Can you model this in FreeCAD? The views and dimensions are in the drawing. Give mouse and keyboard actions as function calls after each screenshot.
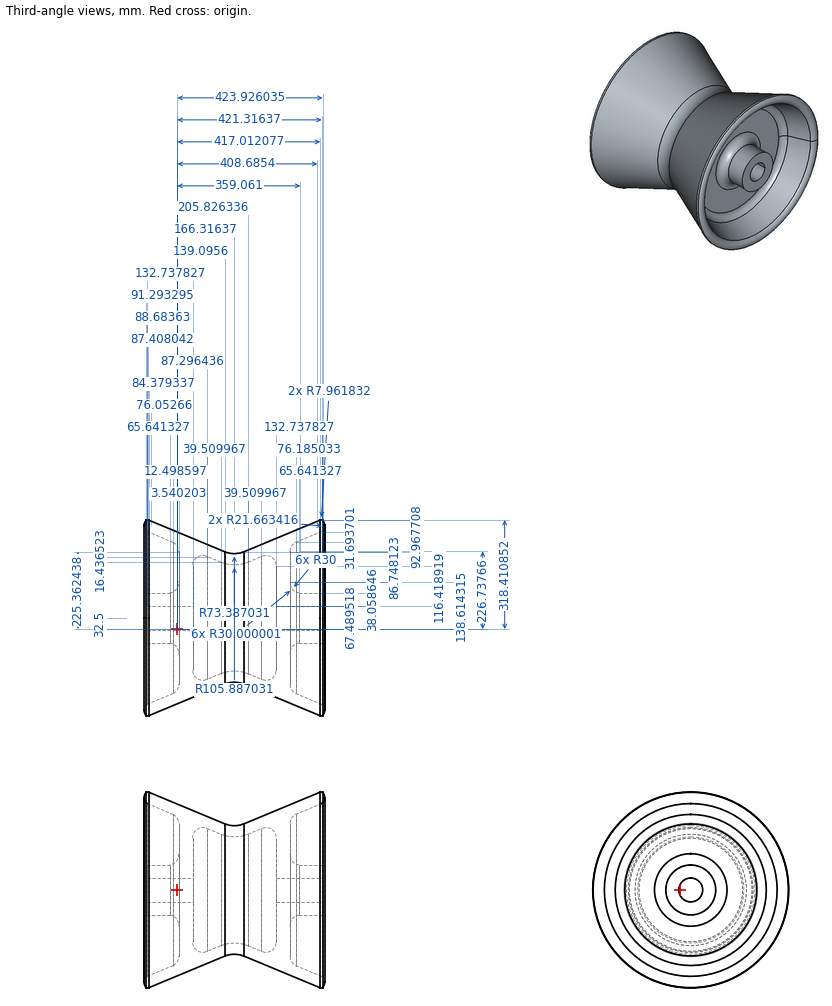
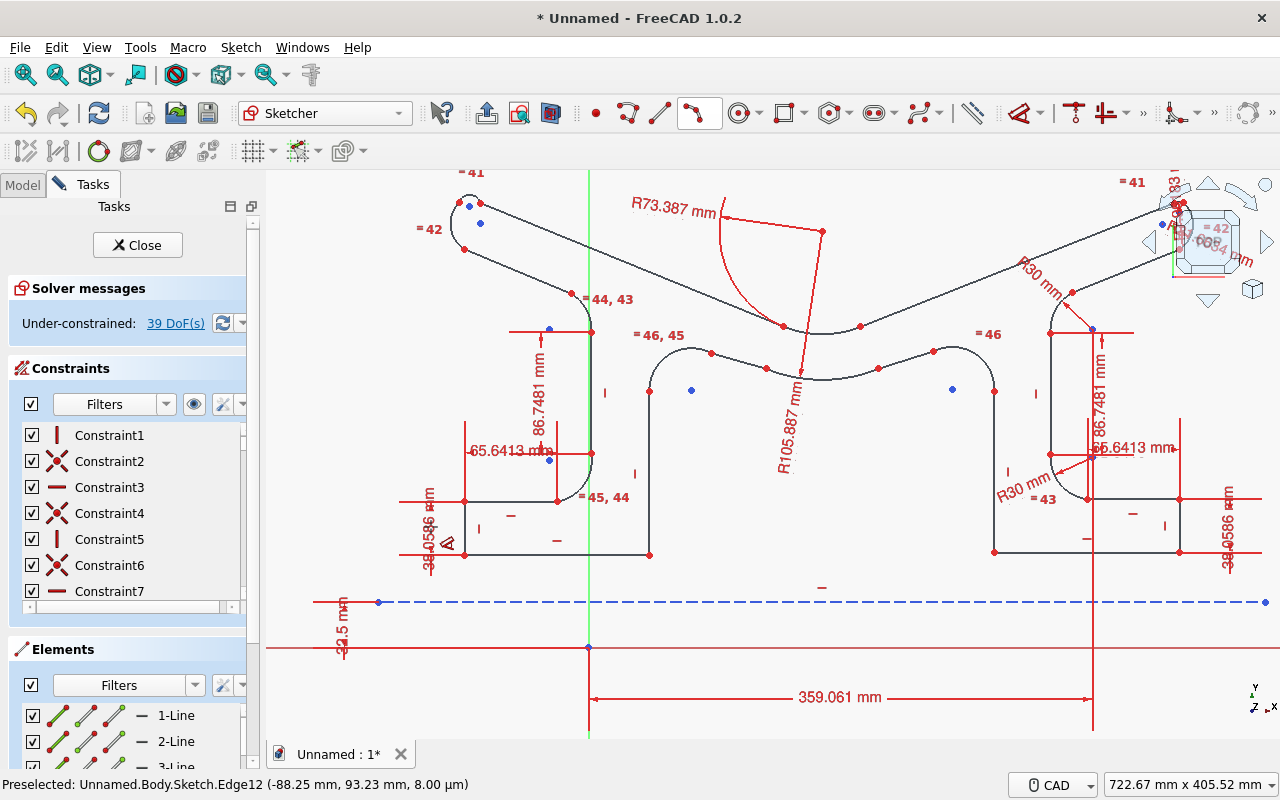
click(783, 326)
click(686, 682)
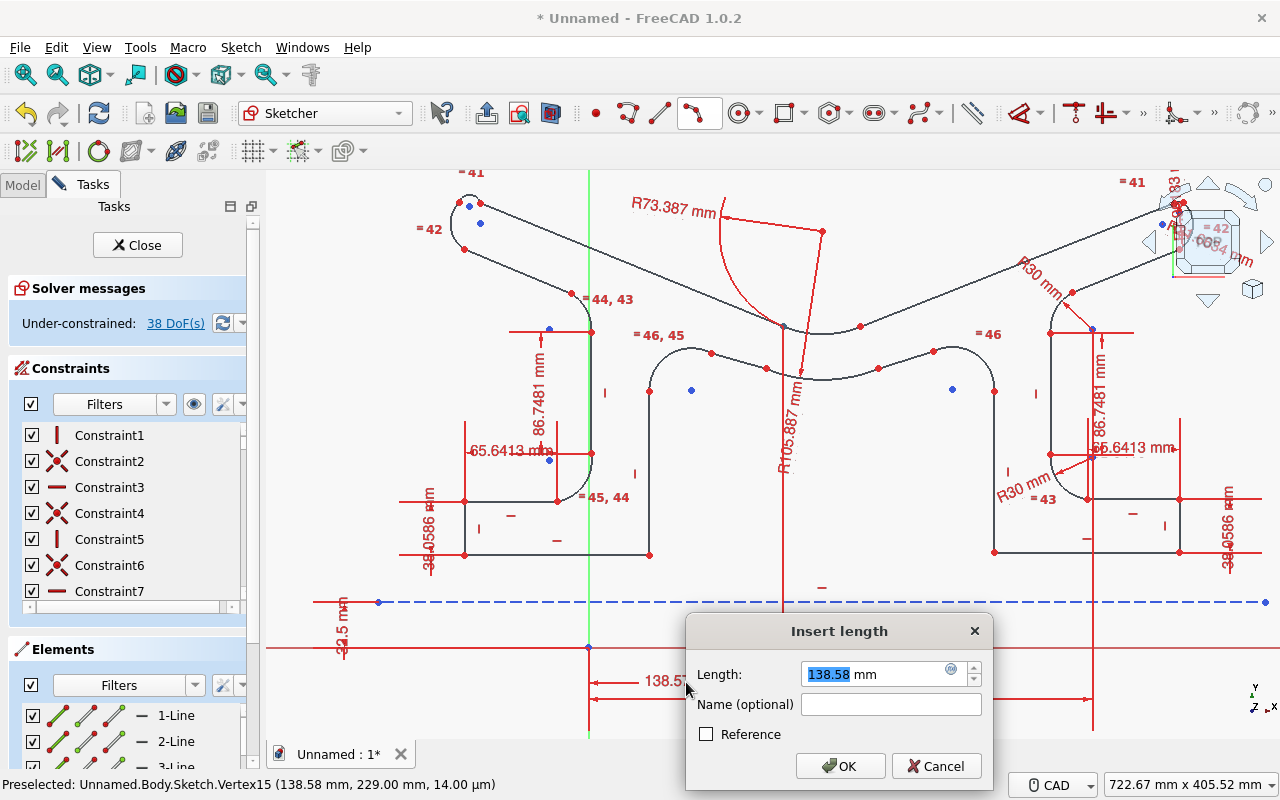
text(139.0956)
key(Return)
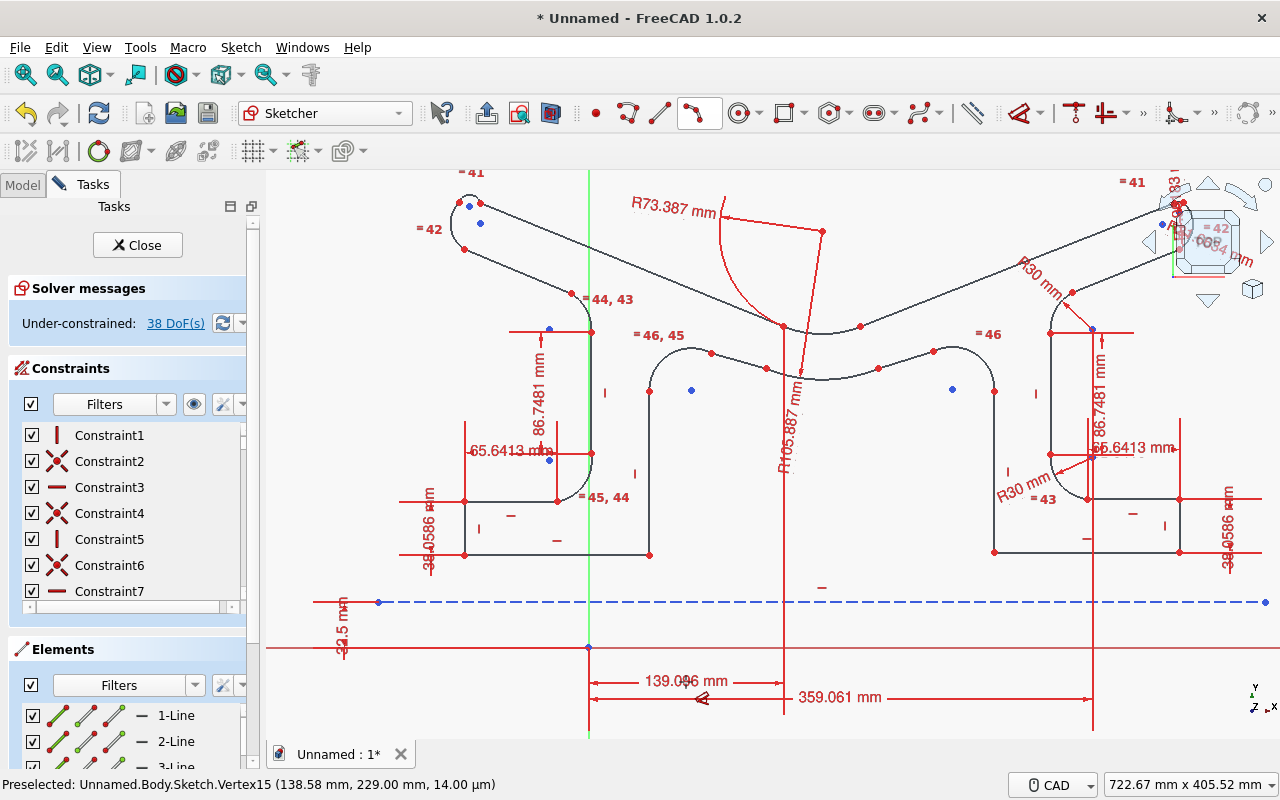
click(464, 249)
click(526, 682)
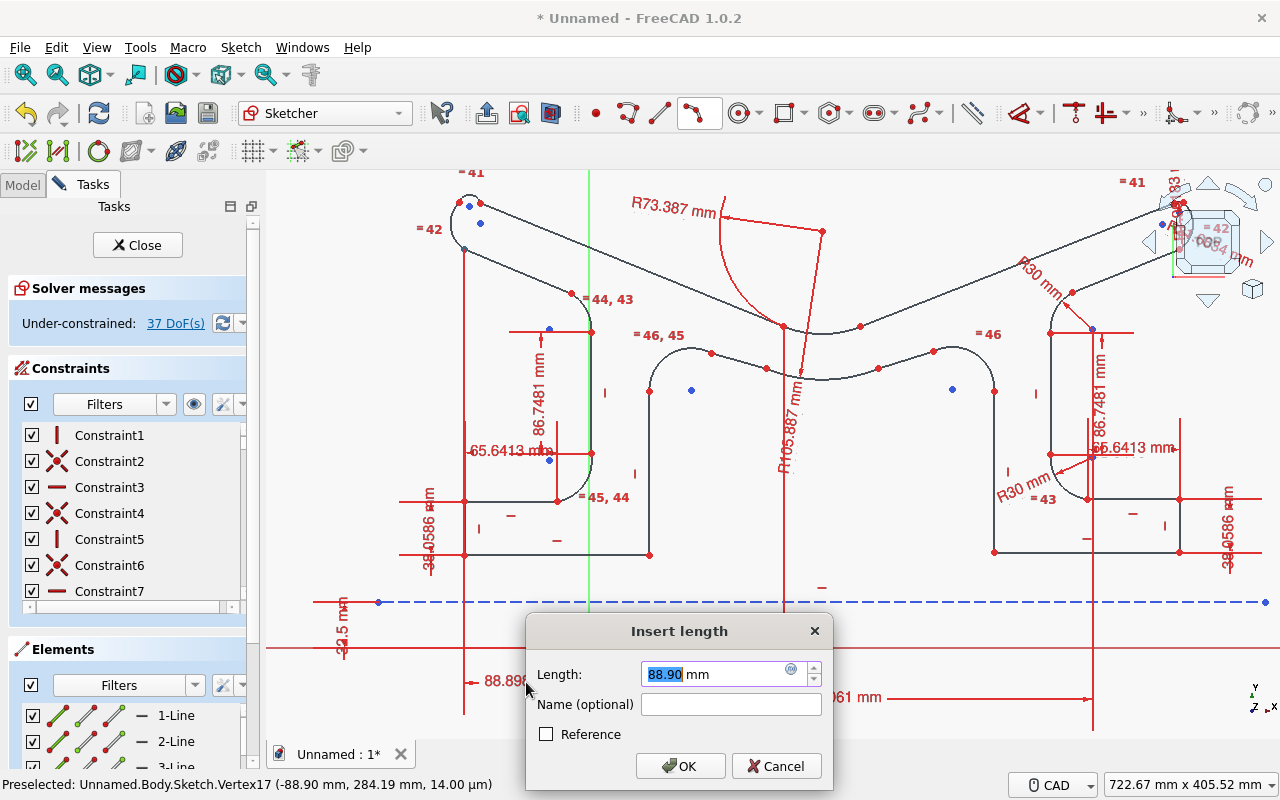
text(88.68363)
key(Return)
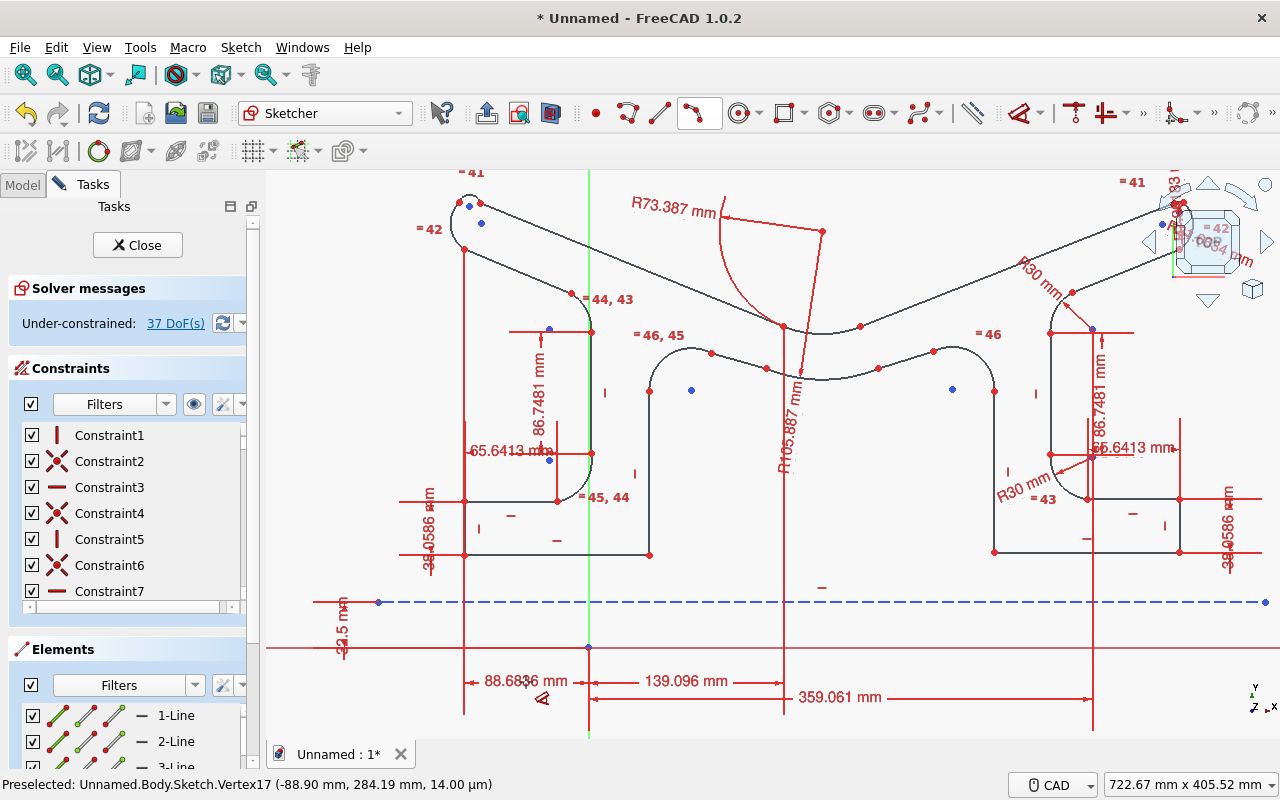
scroll(591, 332, up, 11)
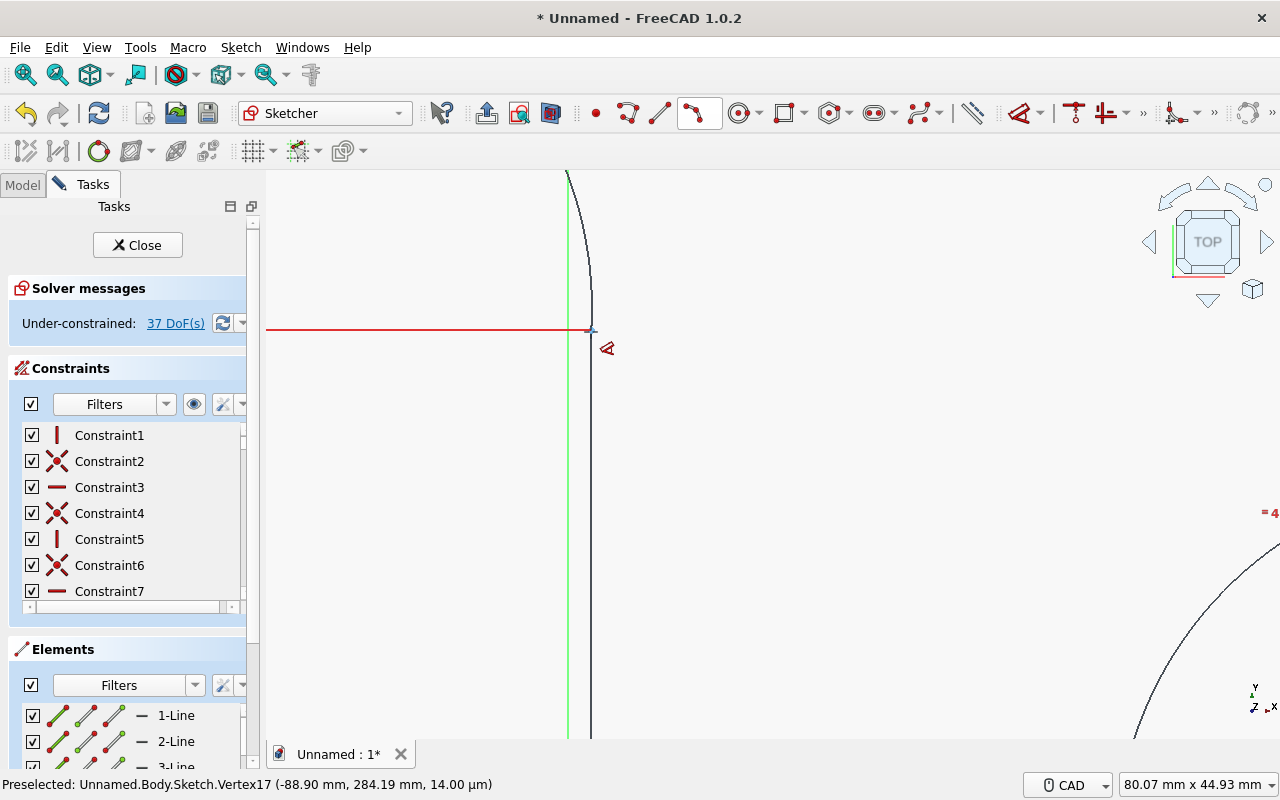
click(591, 330)
click(580, 296)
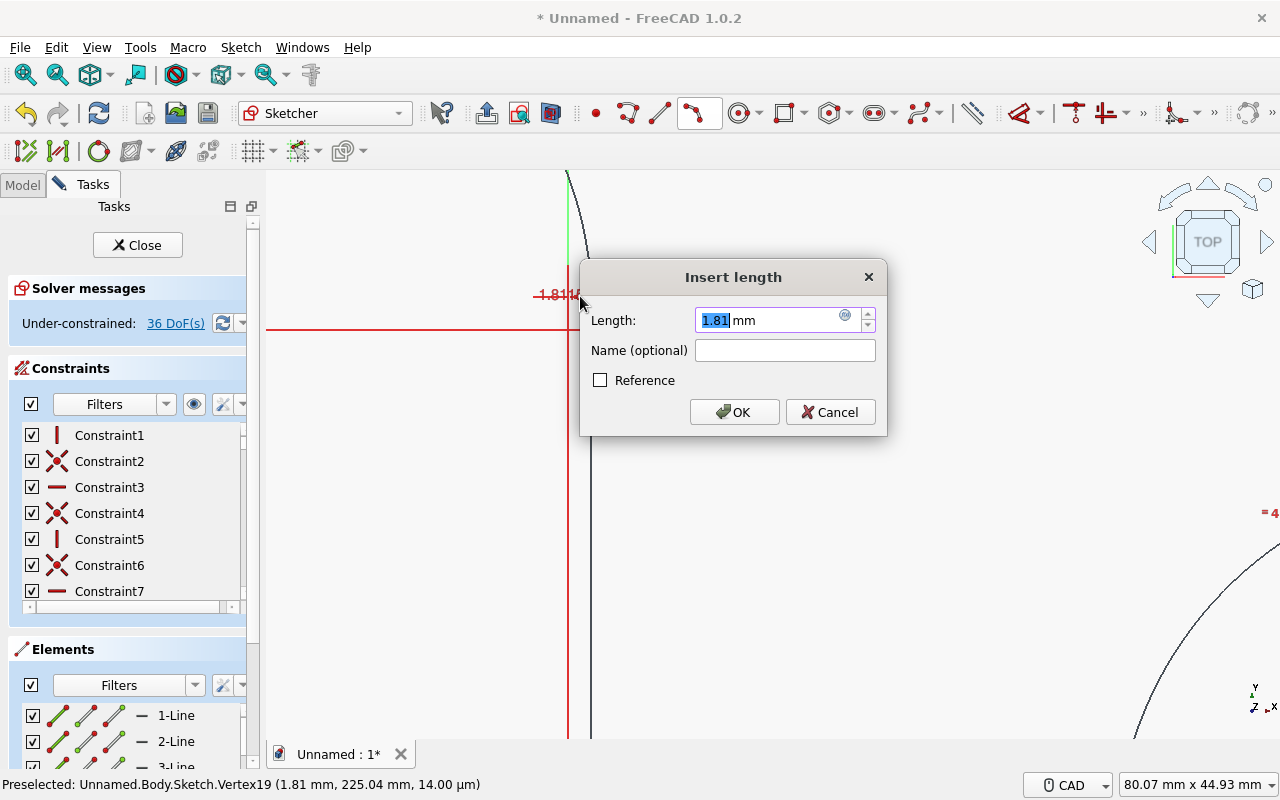
text(3.540203)
key(Return)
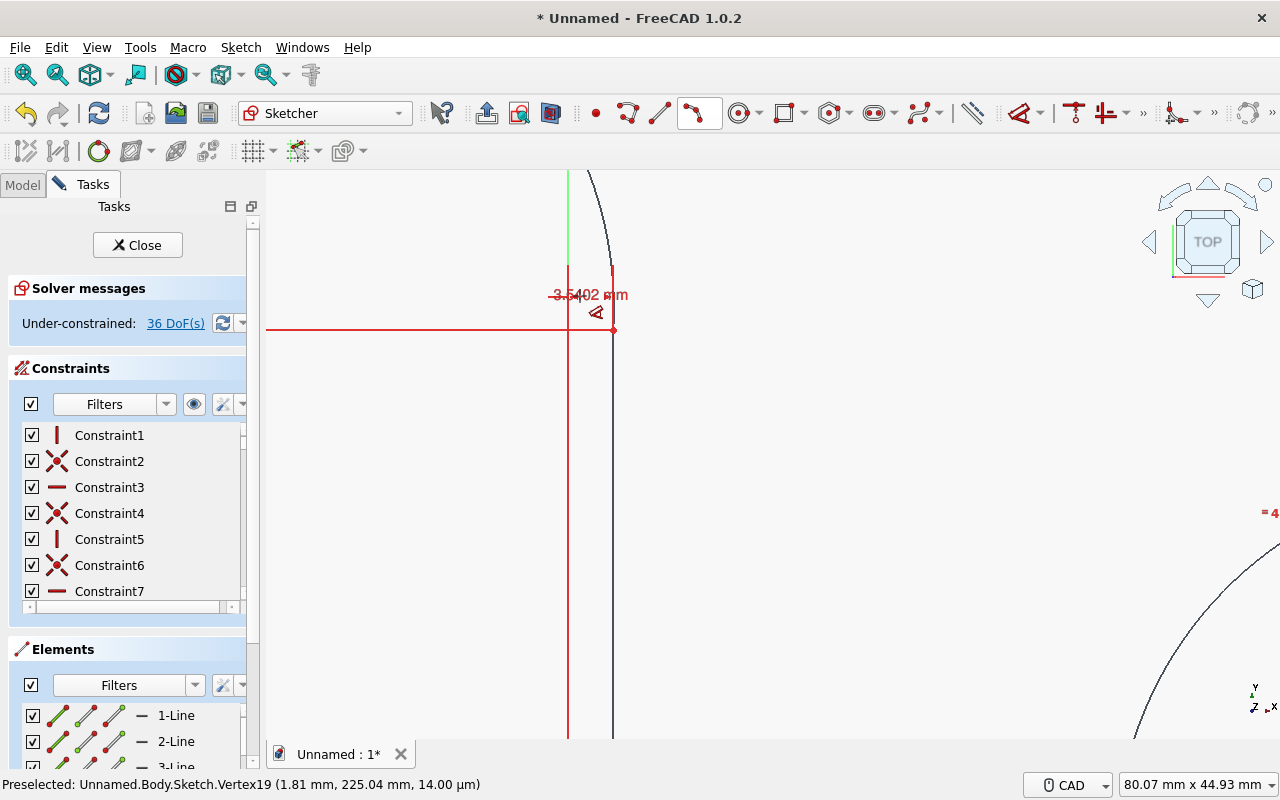
scroll(546, 398, down, 13)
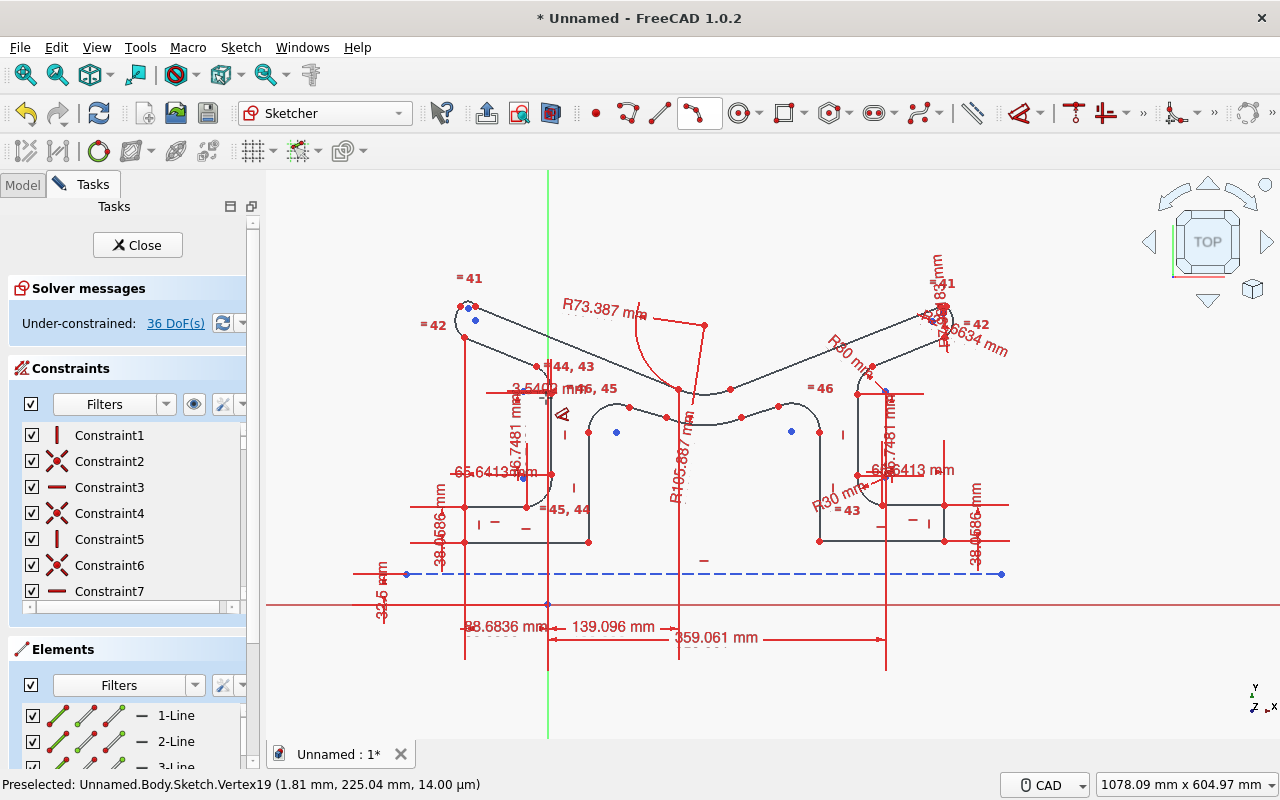
click(465, 507)
click(506, 663)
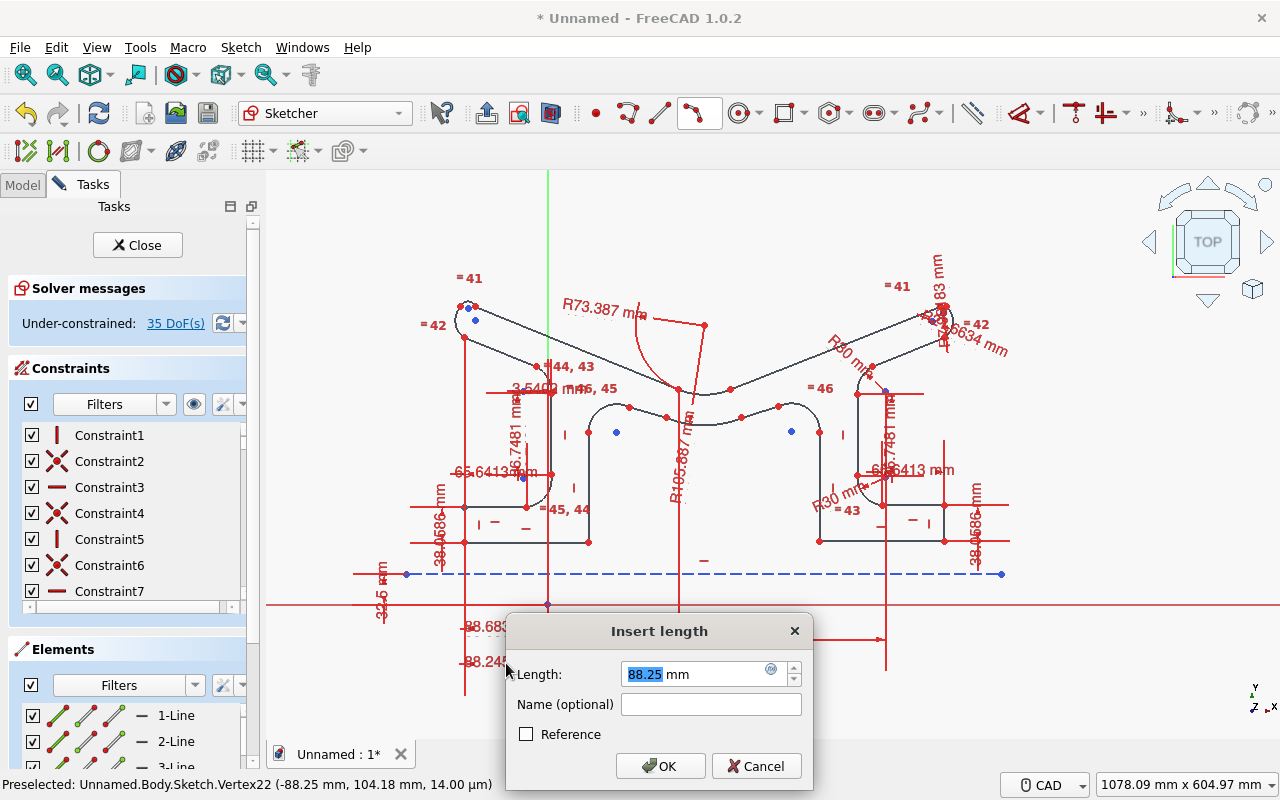
text(88.68363)
key(Return)